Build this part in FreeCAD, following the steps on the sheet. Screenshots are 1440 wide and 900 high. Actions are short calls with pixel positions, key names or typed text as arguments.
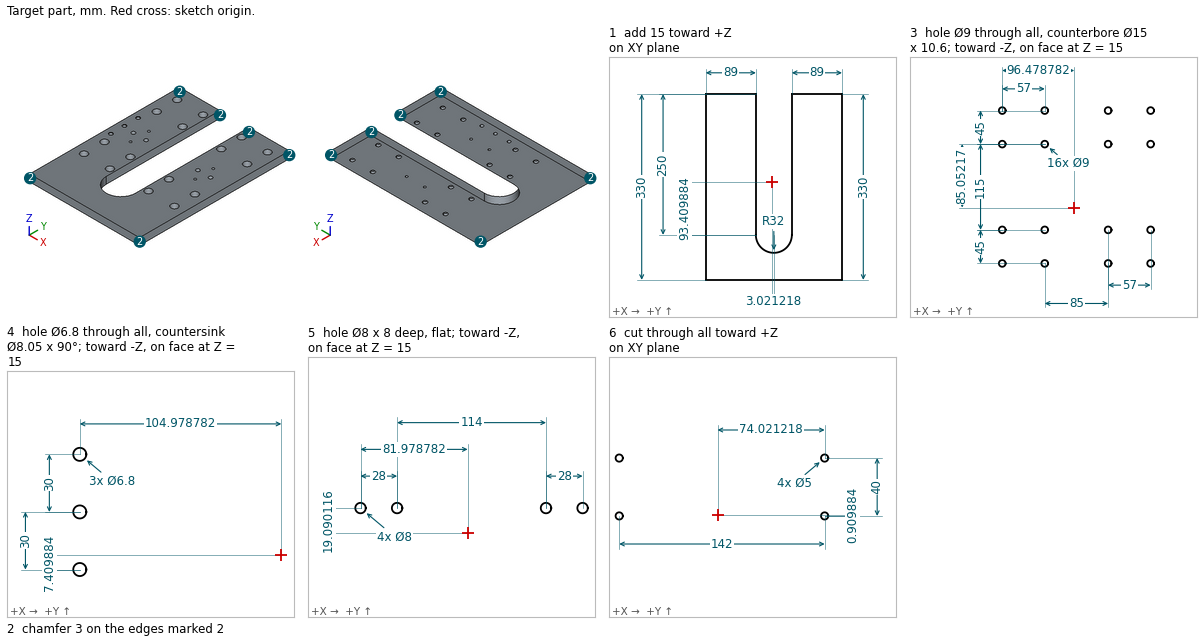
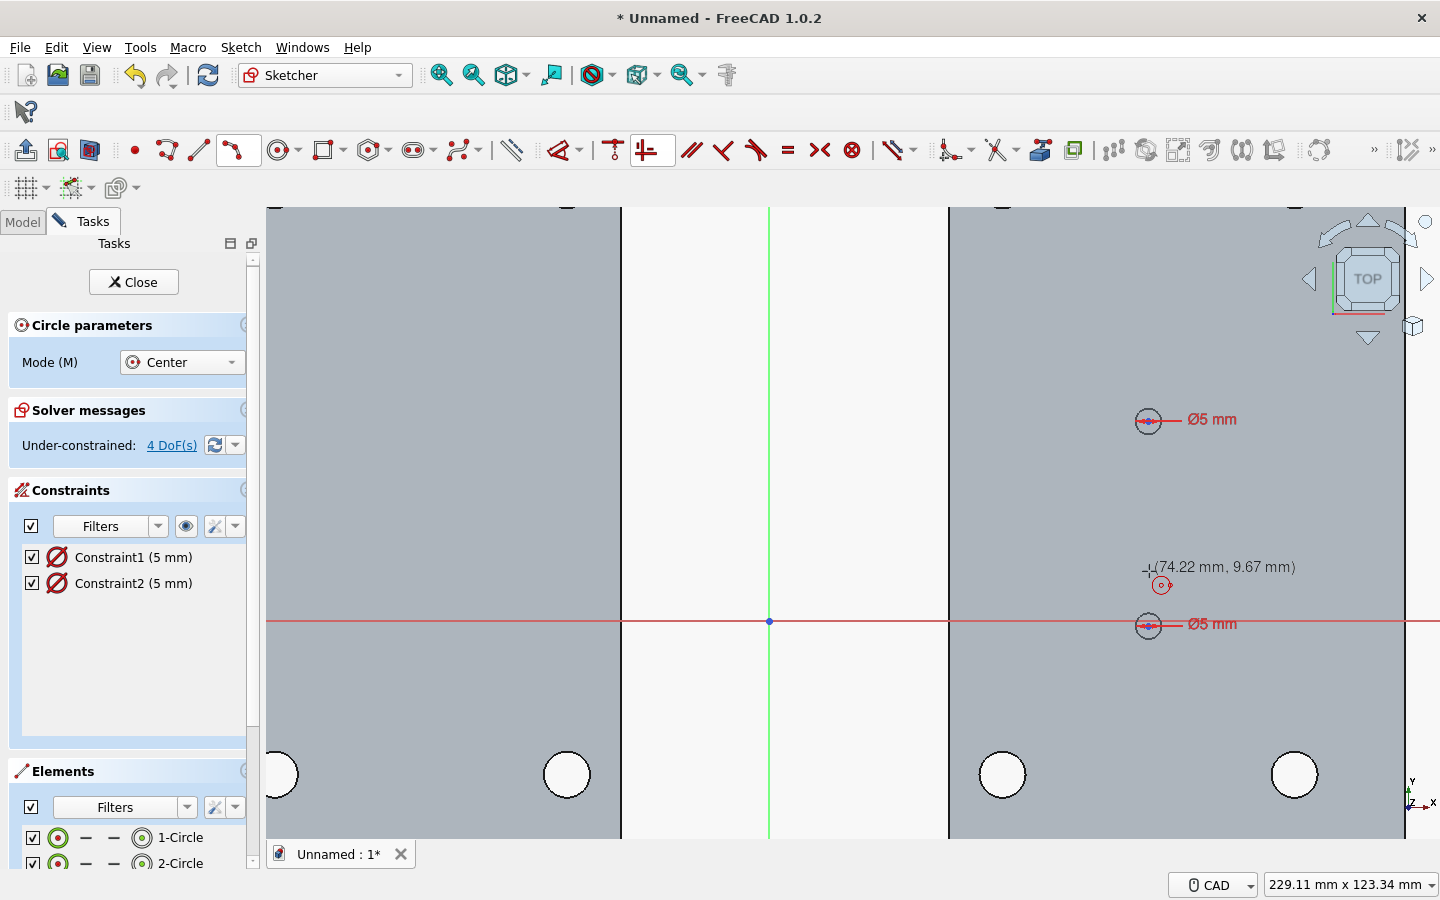
scroll(421, 626, up, 7)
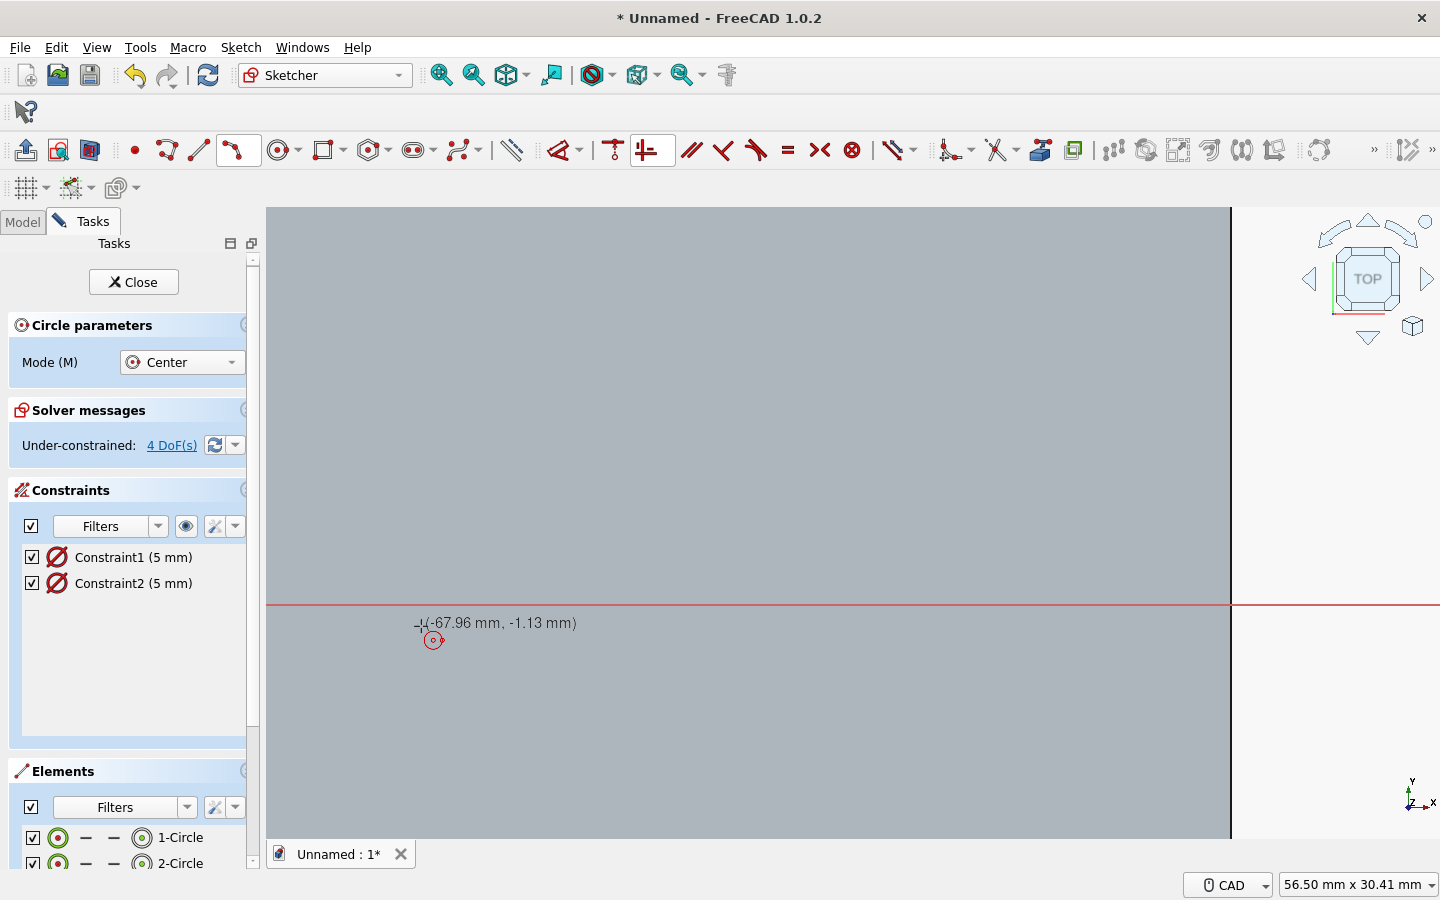
click(420, 624)
move(457, 587)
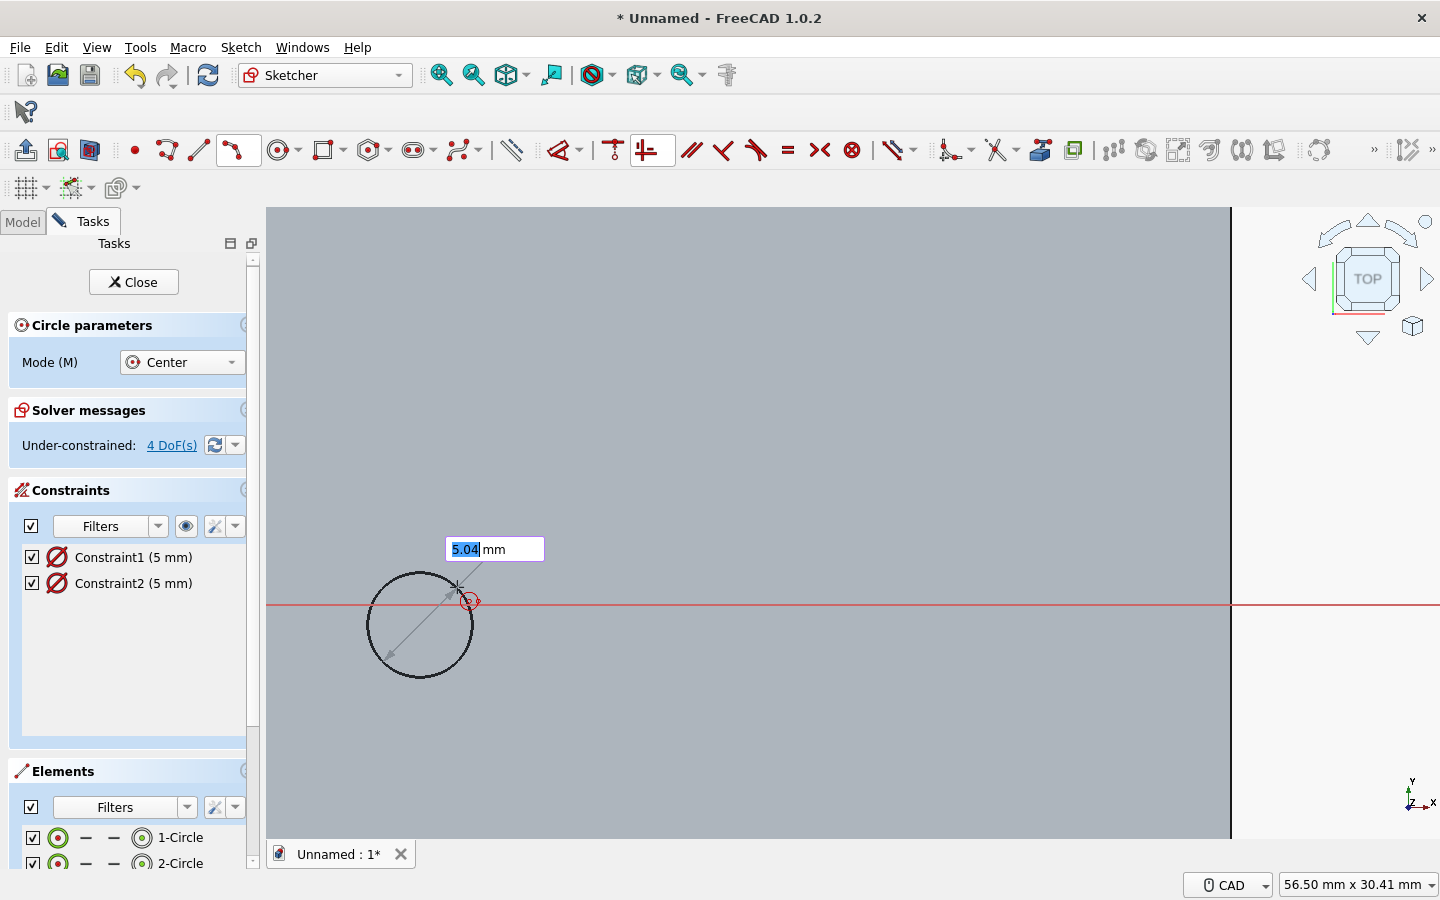
text(5)
key(Return)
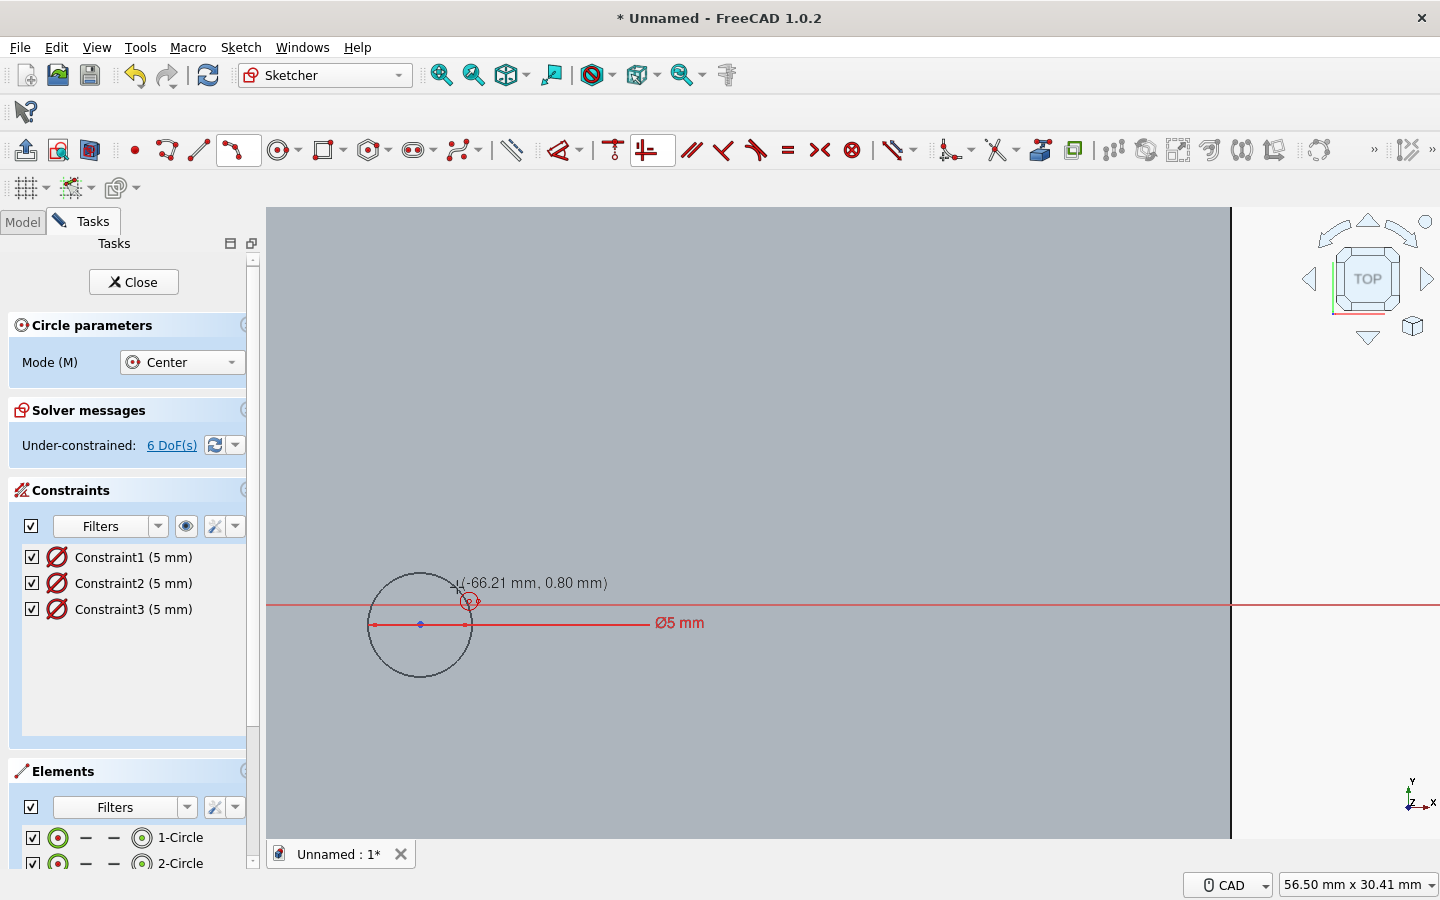
scroll(421, 626, down, 7)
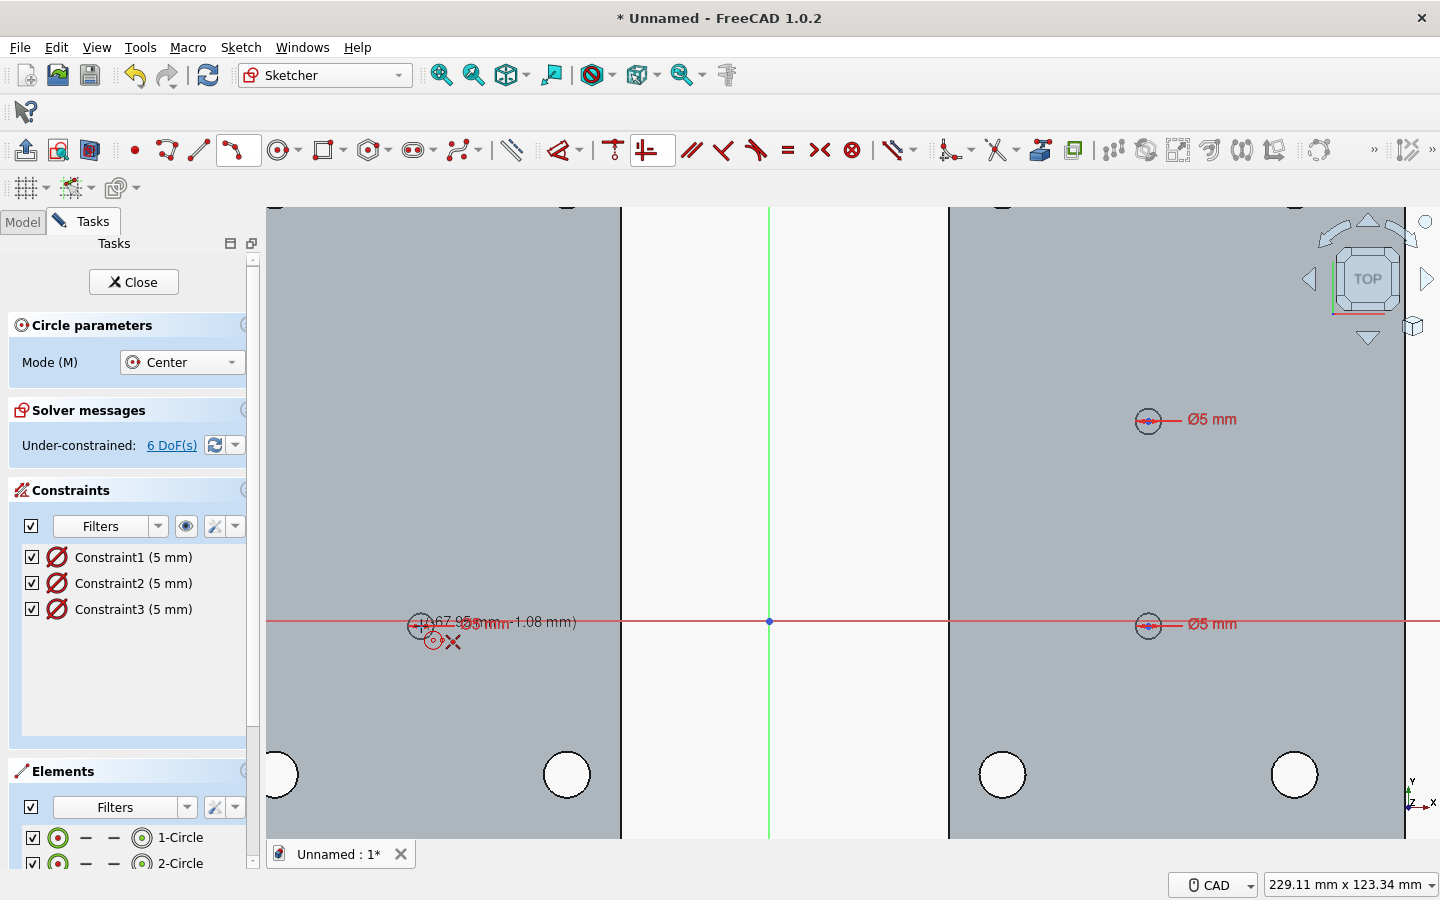
scroll(421, 421, up, 3)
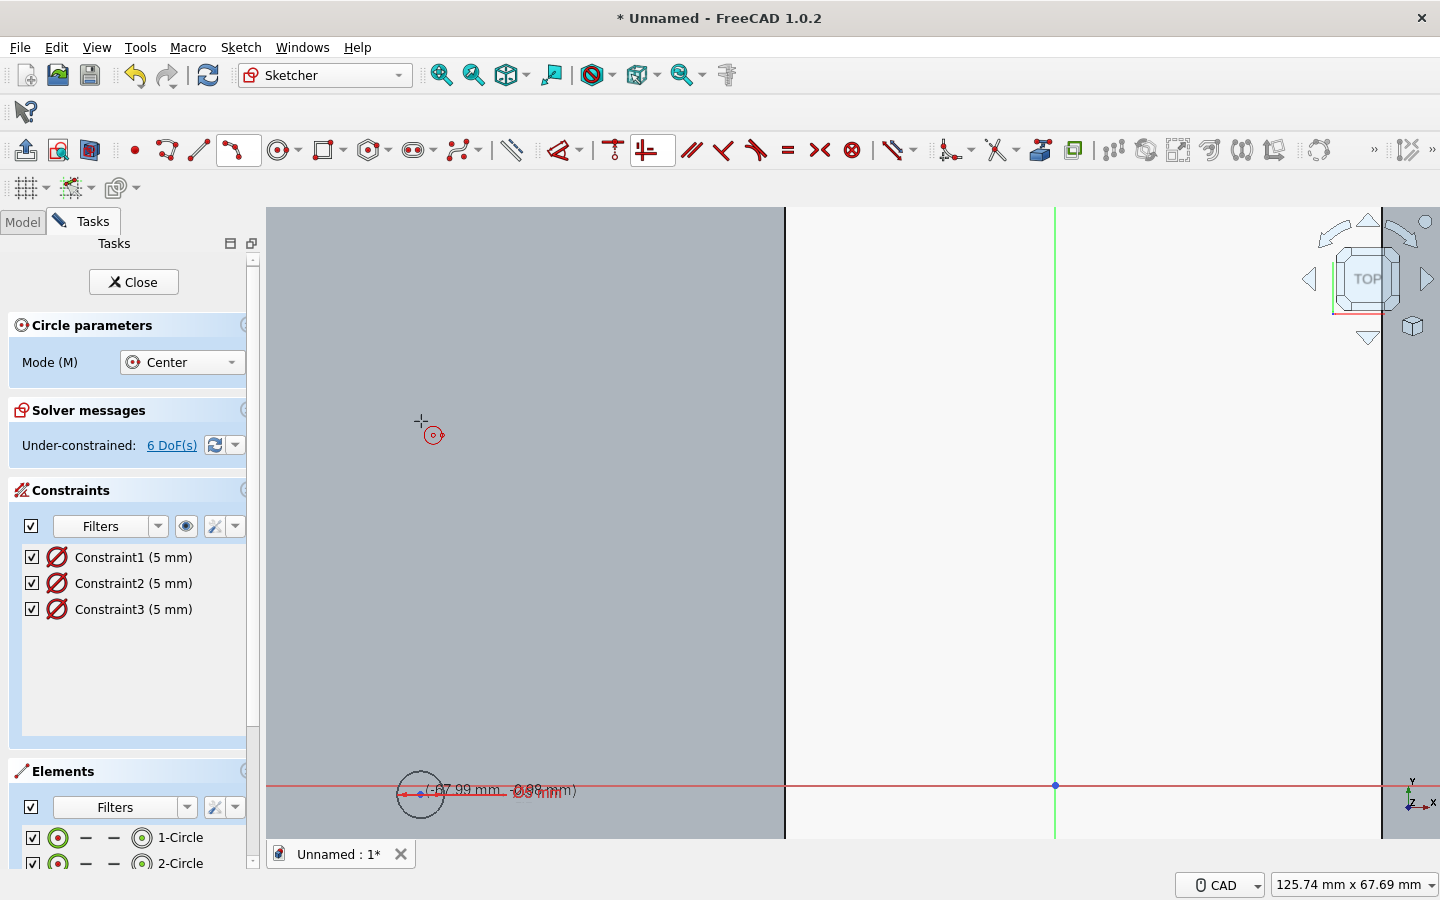
click(421, 421)
move(437, 404)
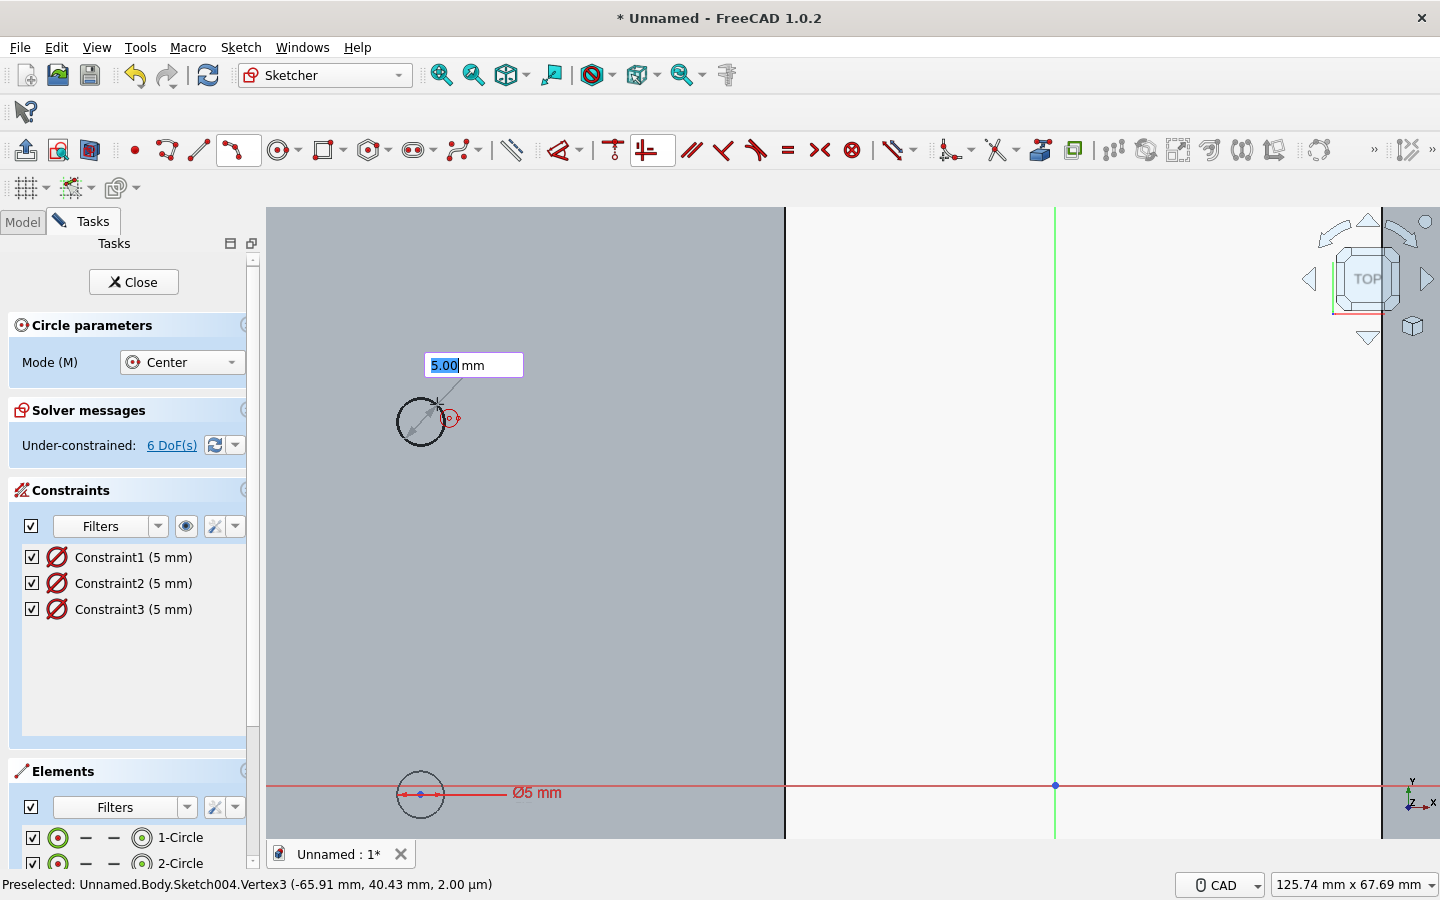
text(5)
key(Return)
key(Escape)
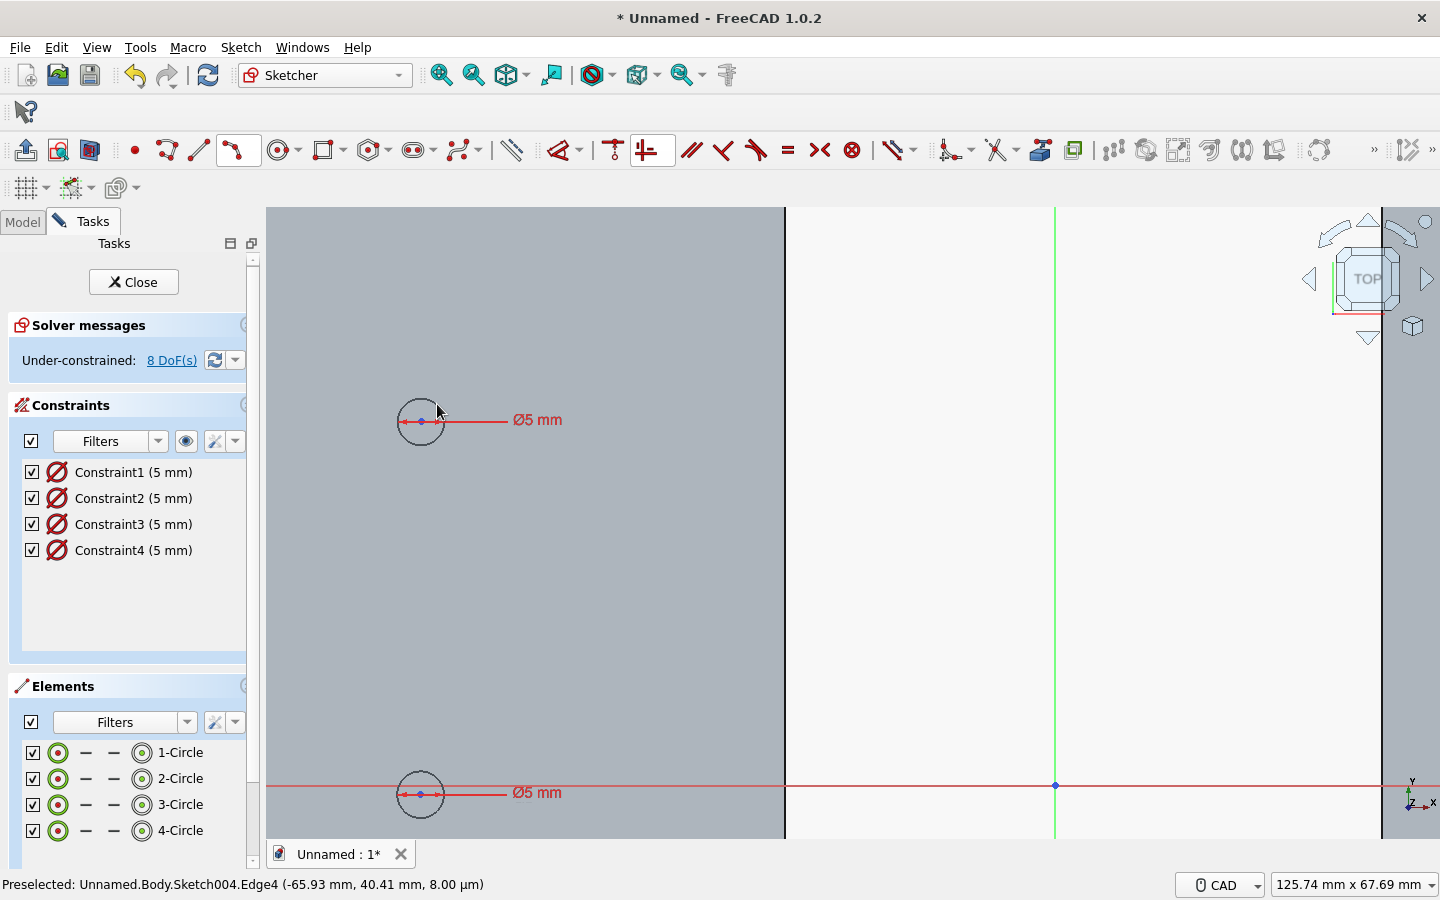
scroll(421, 420, down, 3)